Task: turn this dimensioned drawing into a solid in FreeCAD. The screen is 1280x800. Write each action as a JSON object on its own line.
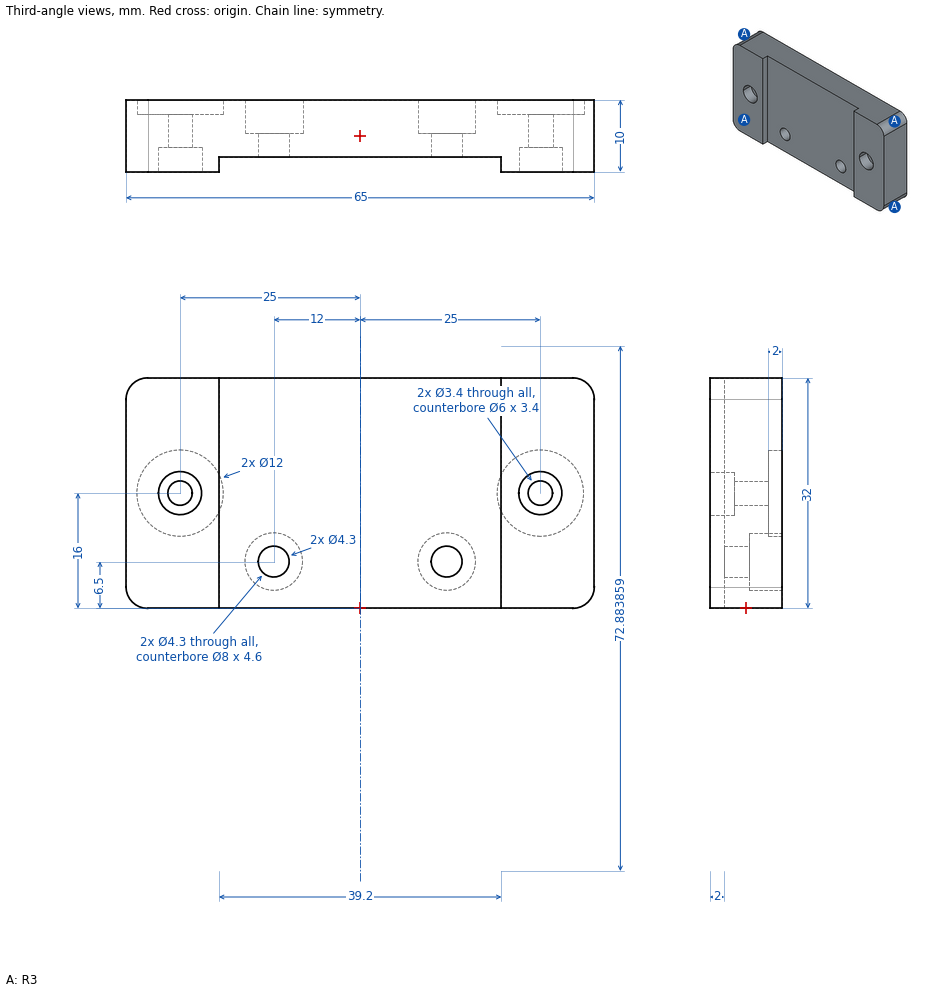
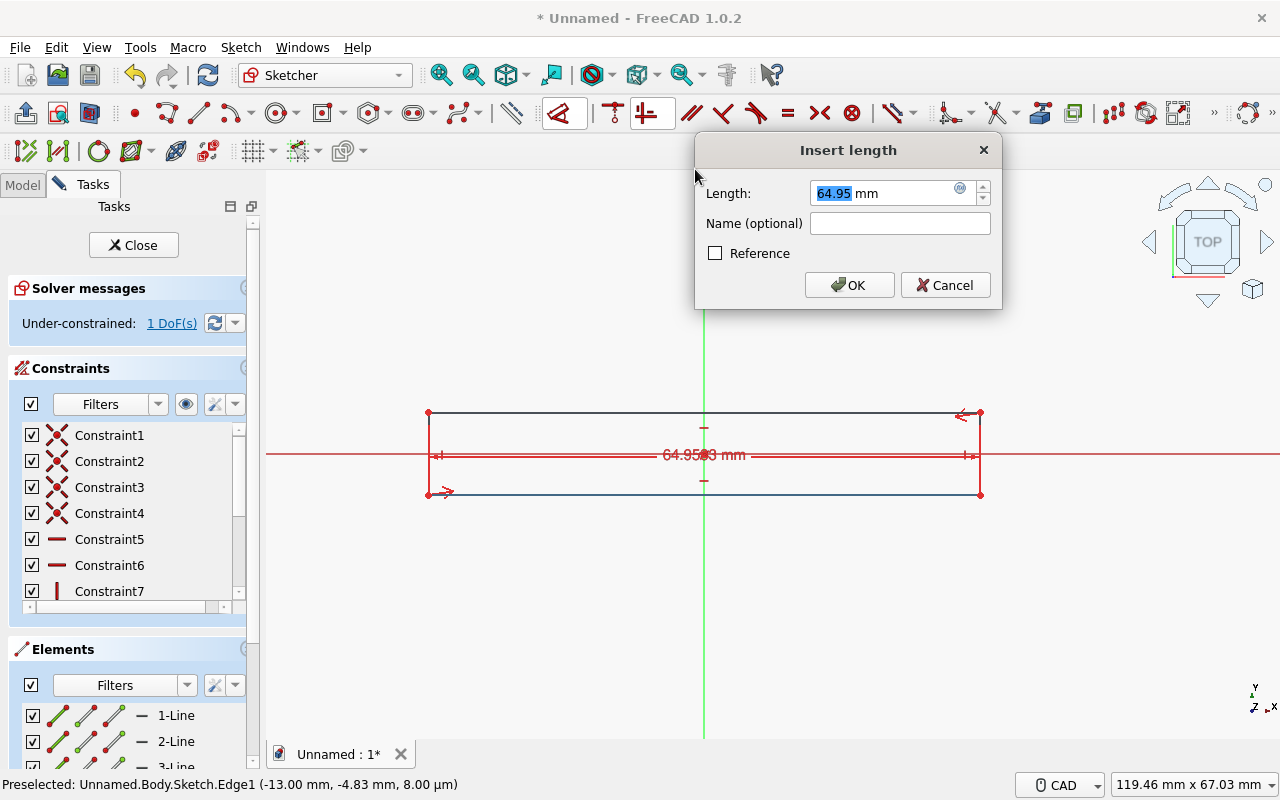
{"action": "type", "text": "65"}
{"action": "key", "text": "Return"}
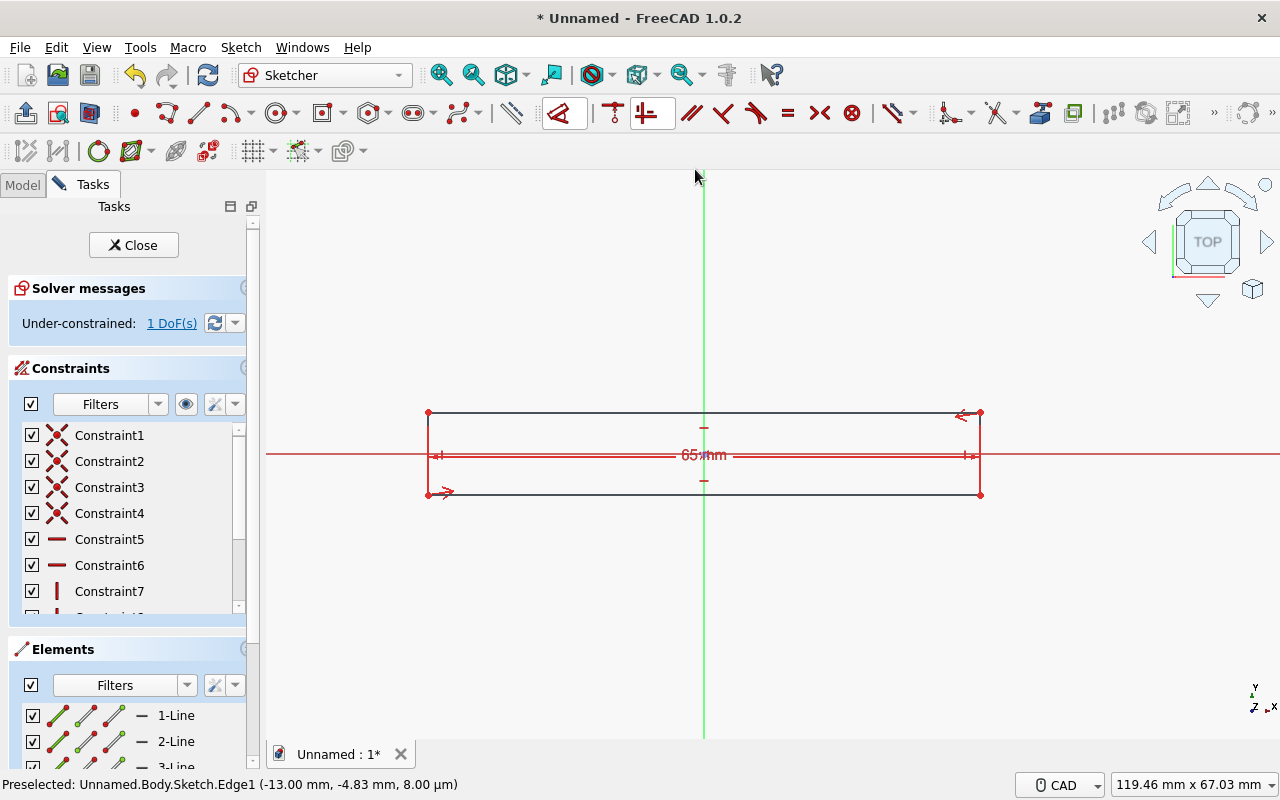
{"action": "left_click", "coordinate": [980, 470]}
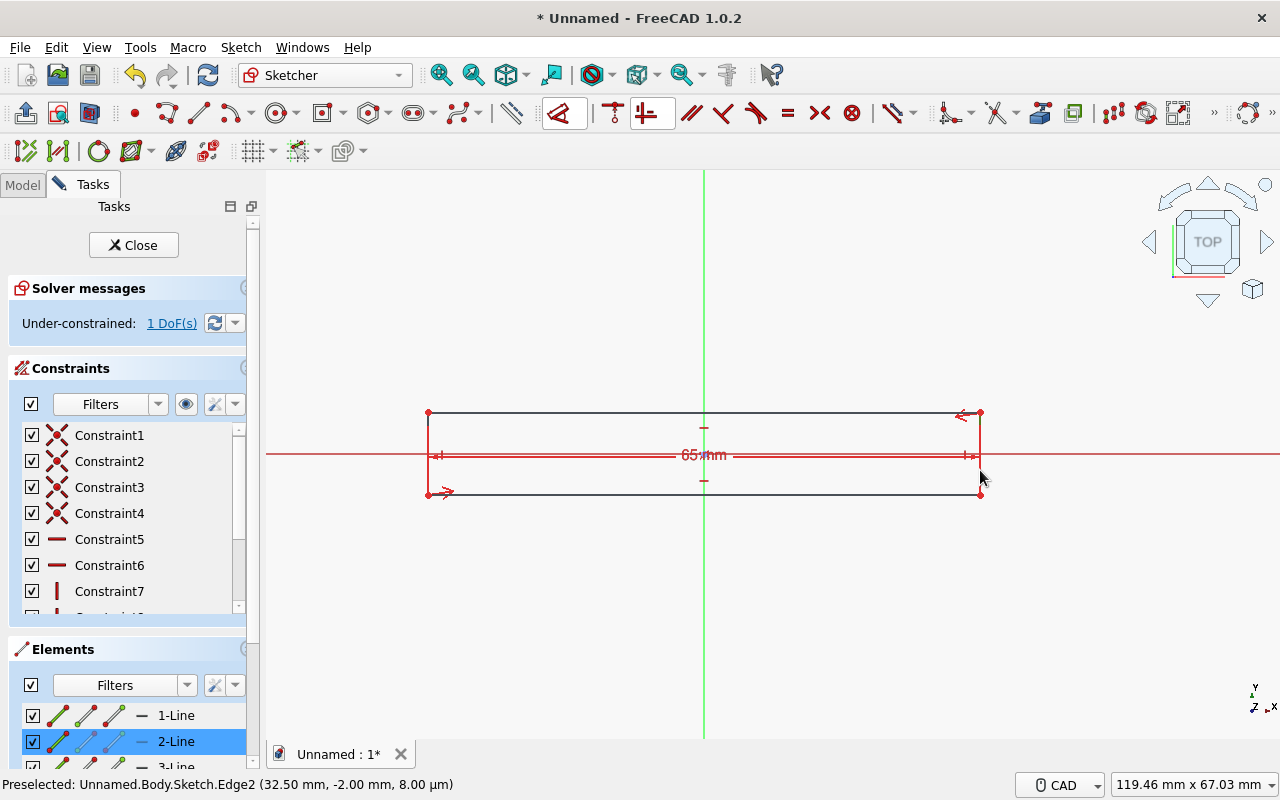
{"action": "left_click", "coordinate": [582, 114]}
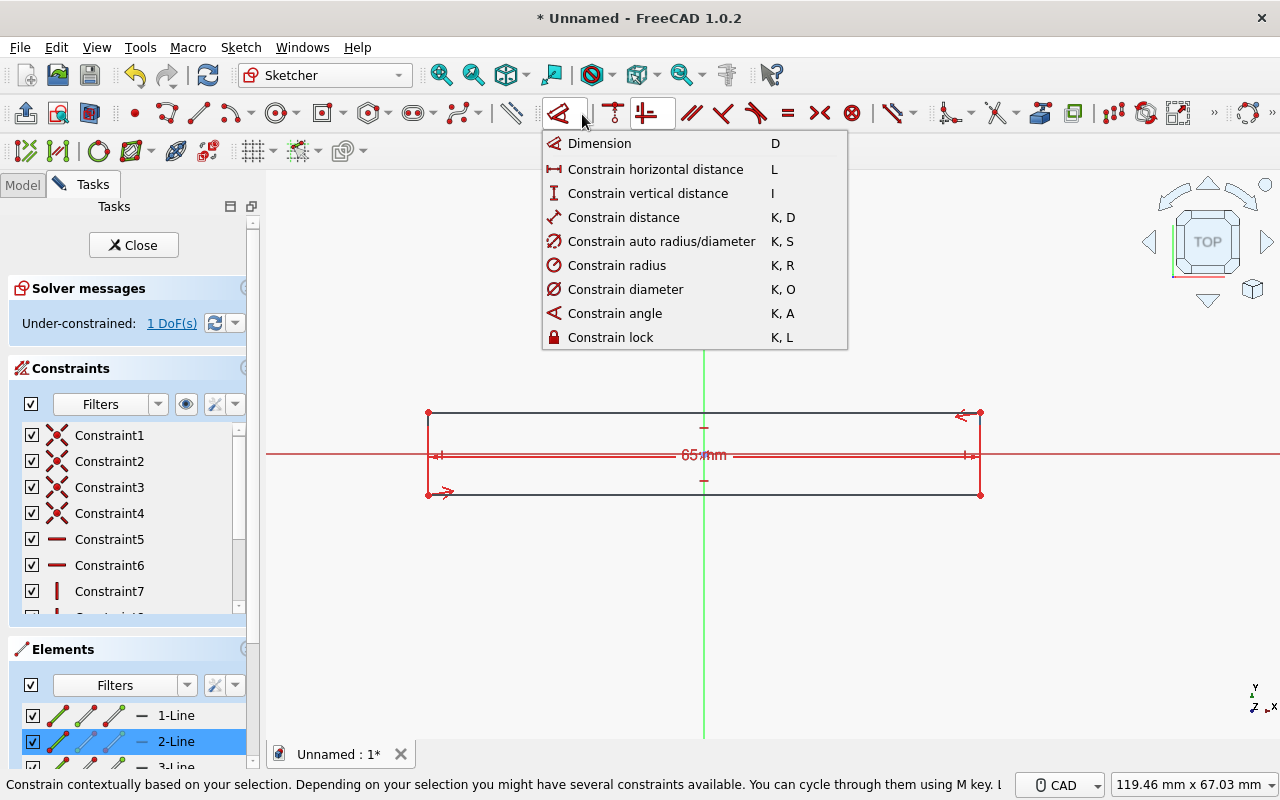
{"action": "left_click", "coordinate": [695, 193]}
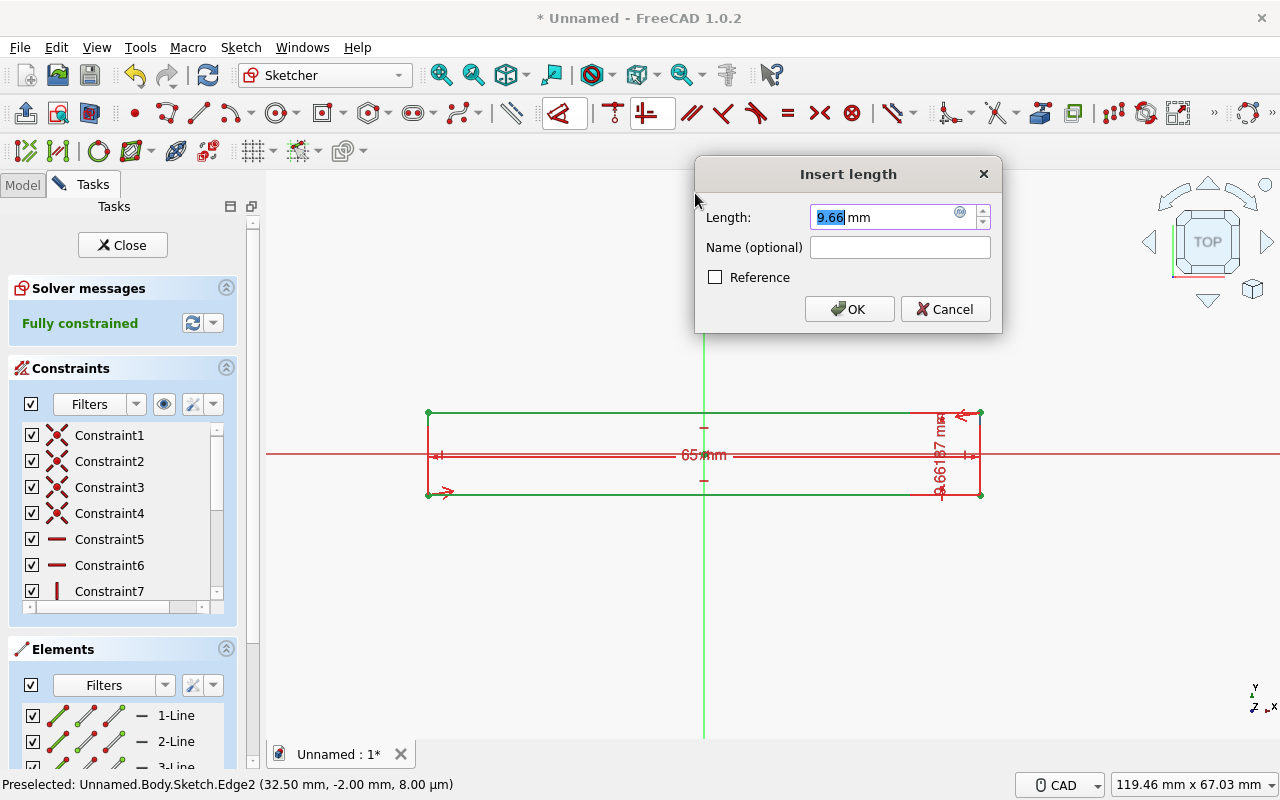
{"action": "type", "text": "10"}
{"action": "key", "text": "Return"}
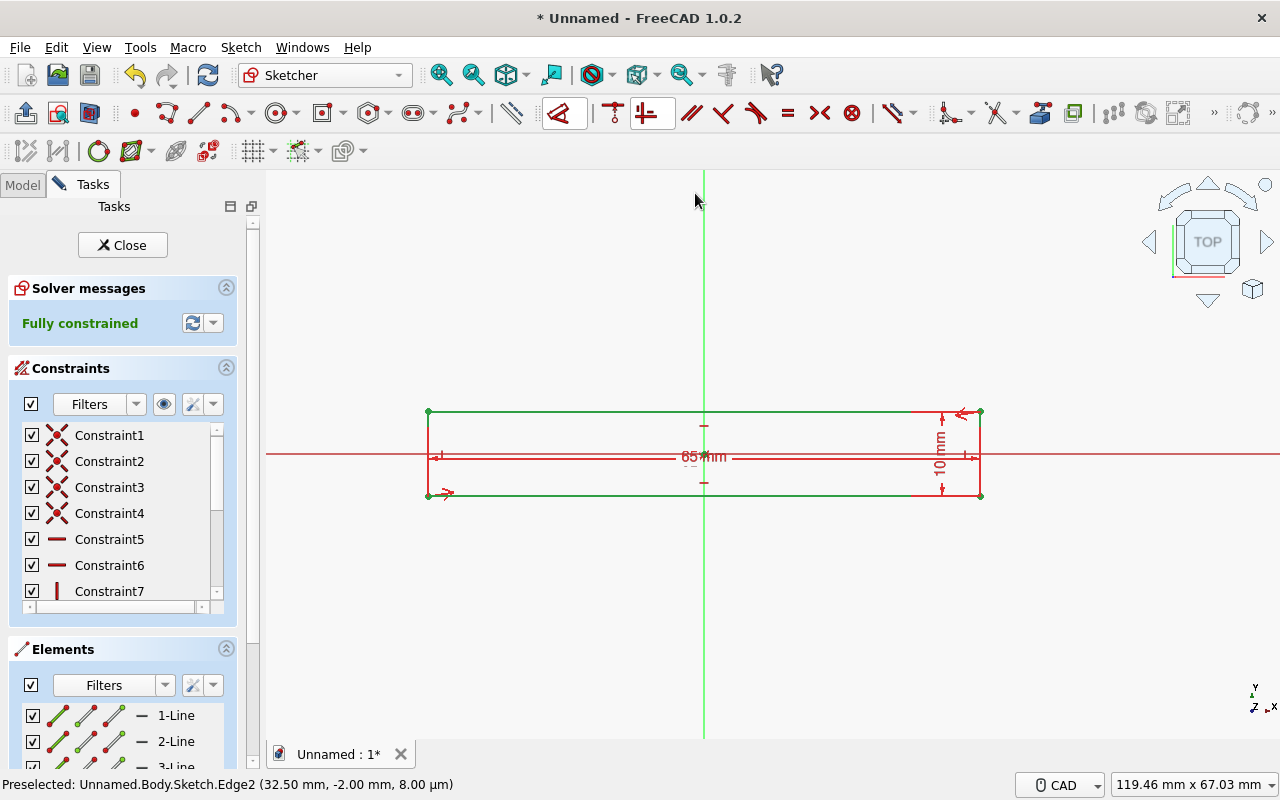
{"action": "left_click", "coordinate": [123, 245]}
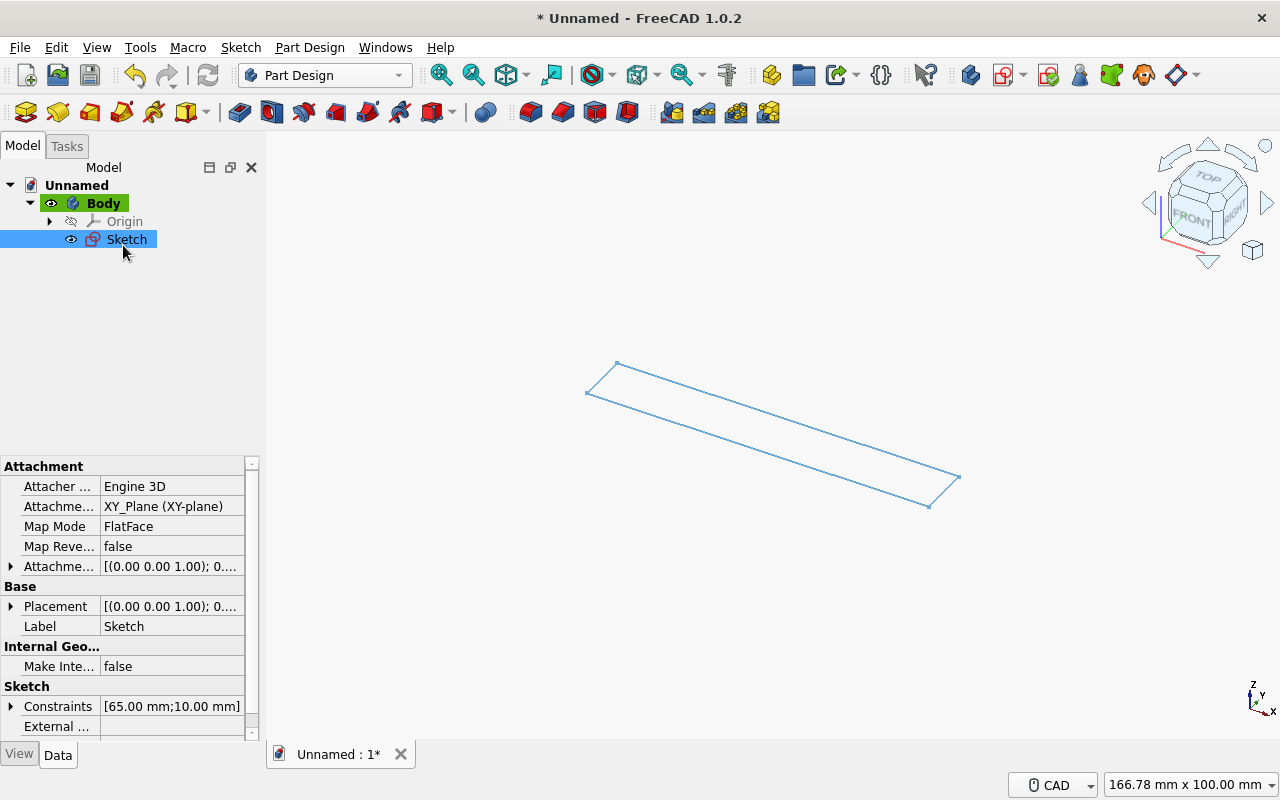
{"action": "left_click", "coordinate": [26, 112]}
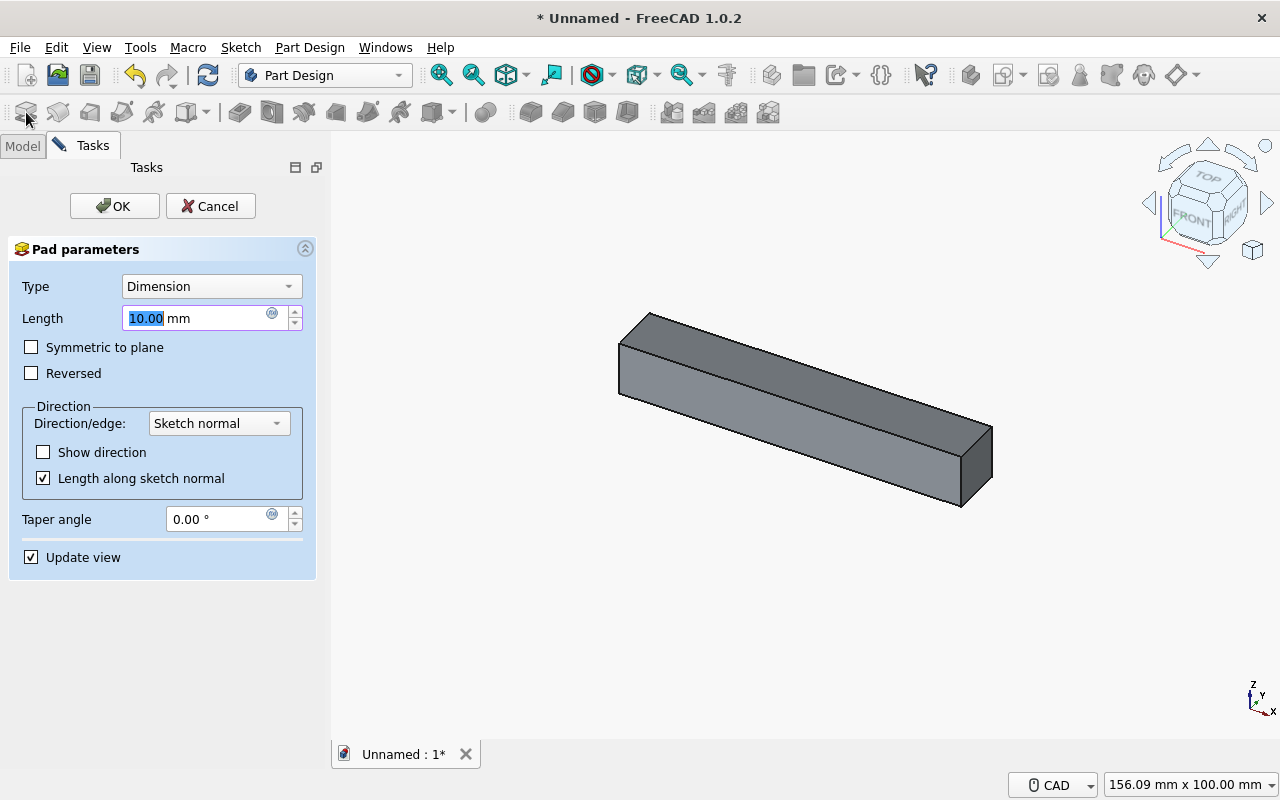
{"action": "type", "text": "32"}
{"action": "key", "text": "Tab"}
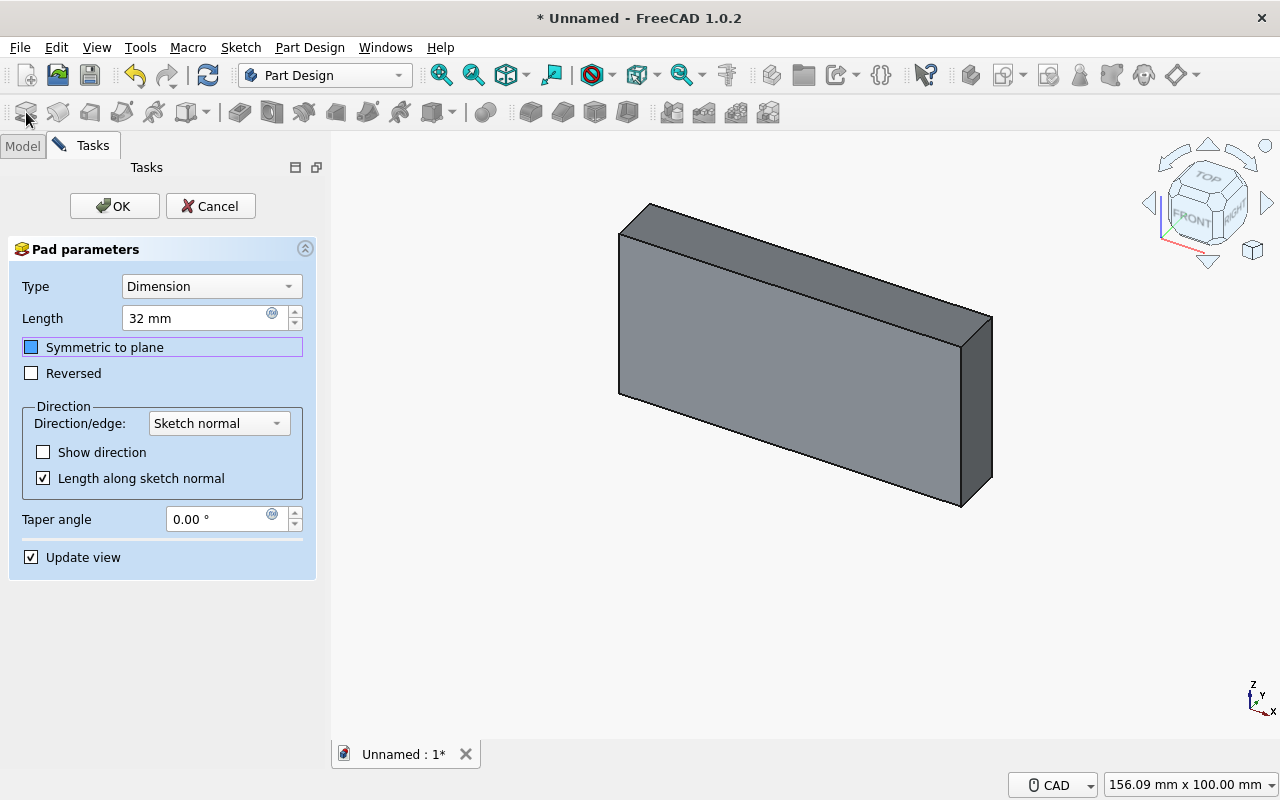
{"action": "left_click", "coordinate": [115, 206]}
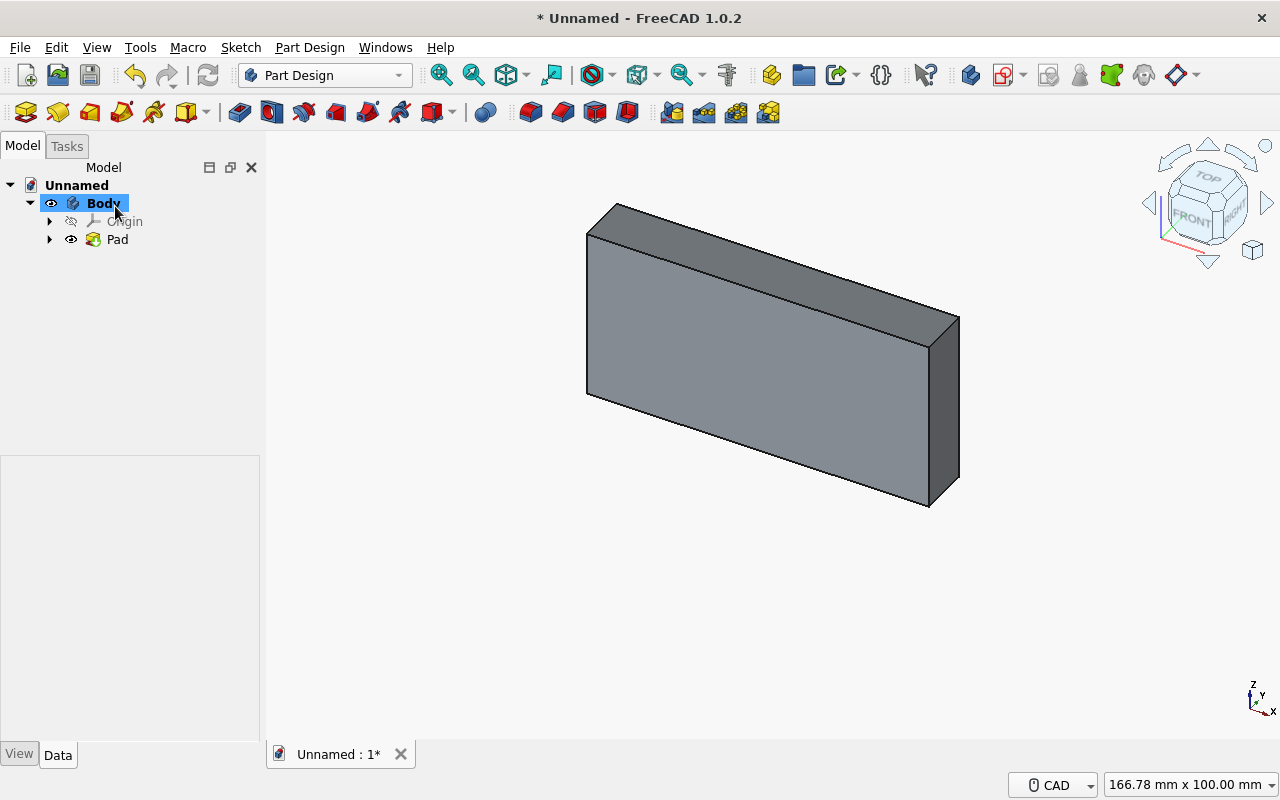
{"action": "left_click", "coordinate": [807, 386]}